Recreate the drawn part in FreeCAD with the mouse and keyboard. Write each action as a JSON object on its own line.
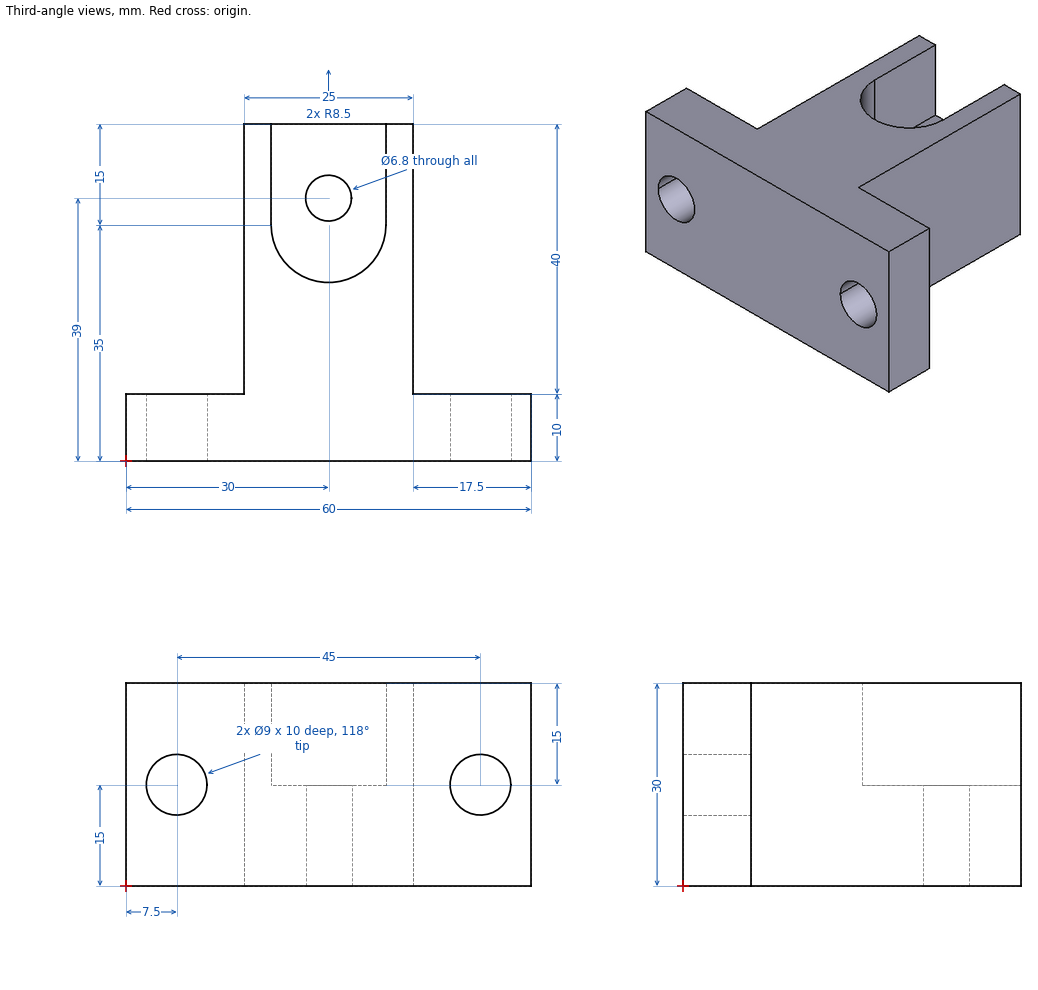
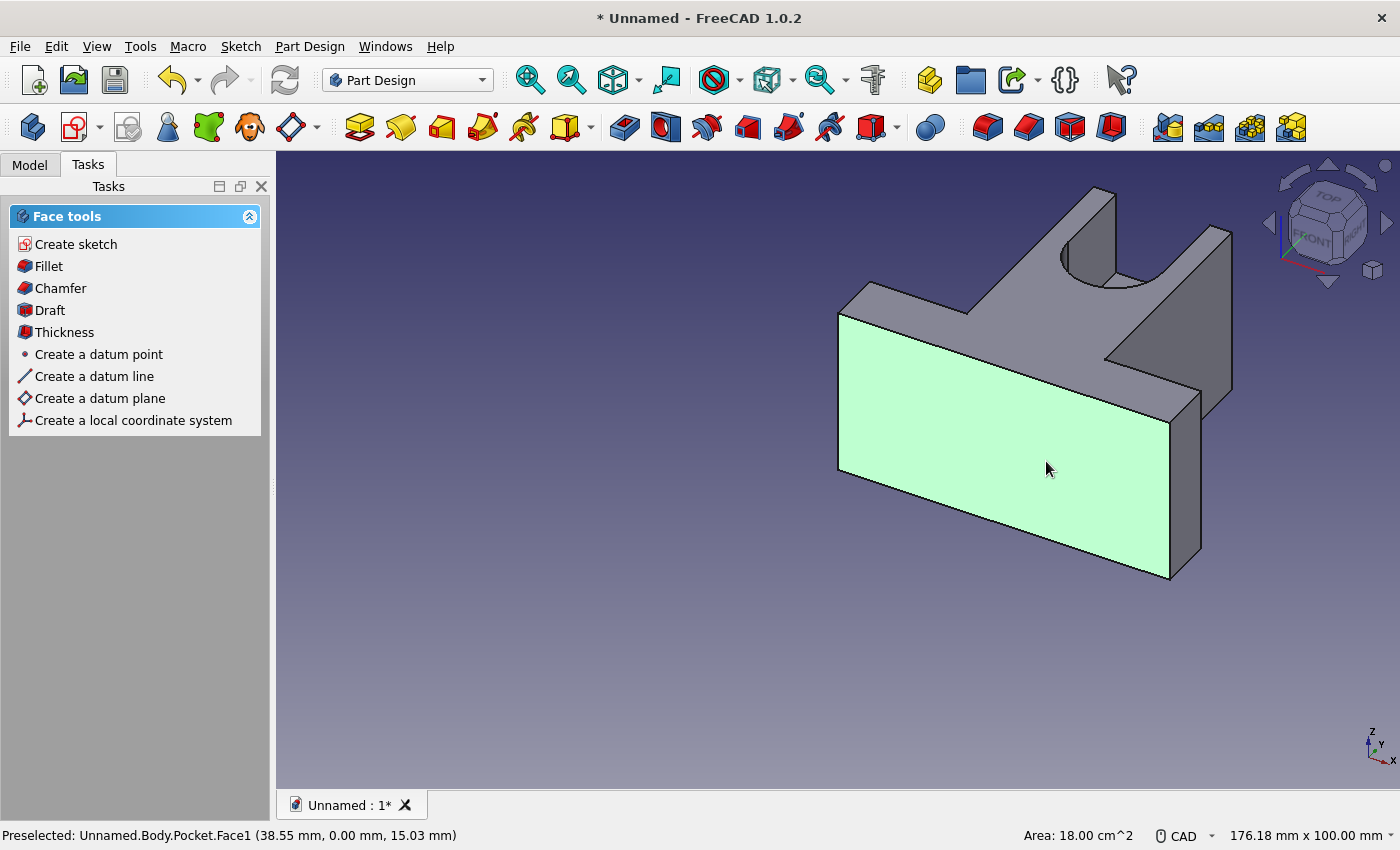
{"action": "left_click", "coordinate": [74, 128]}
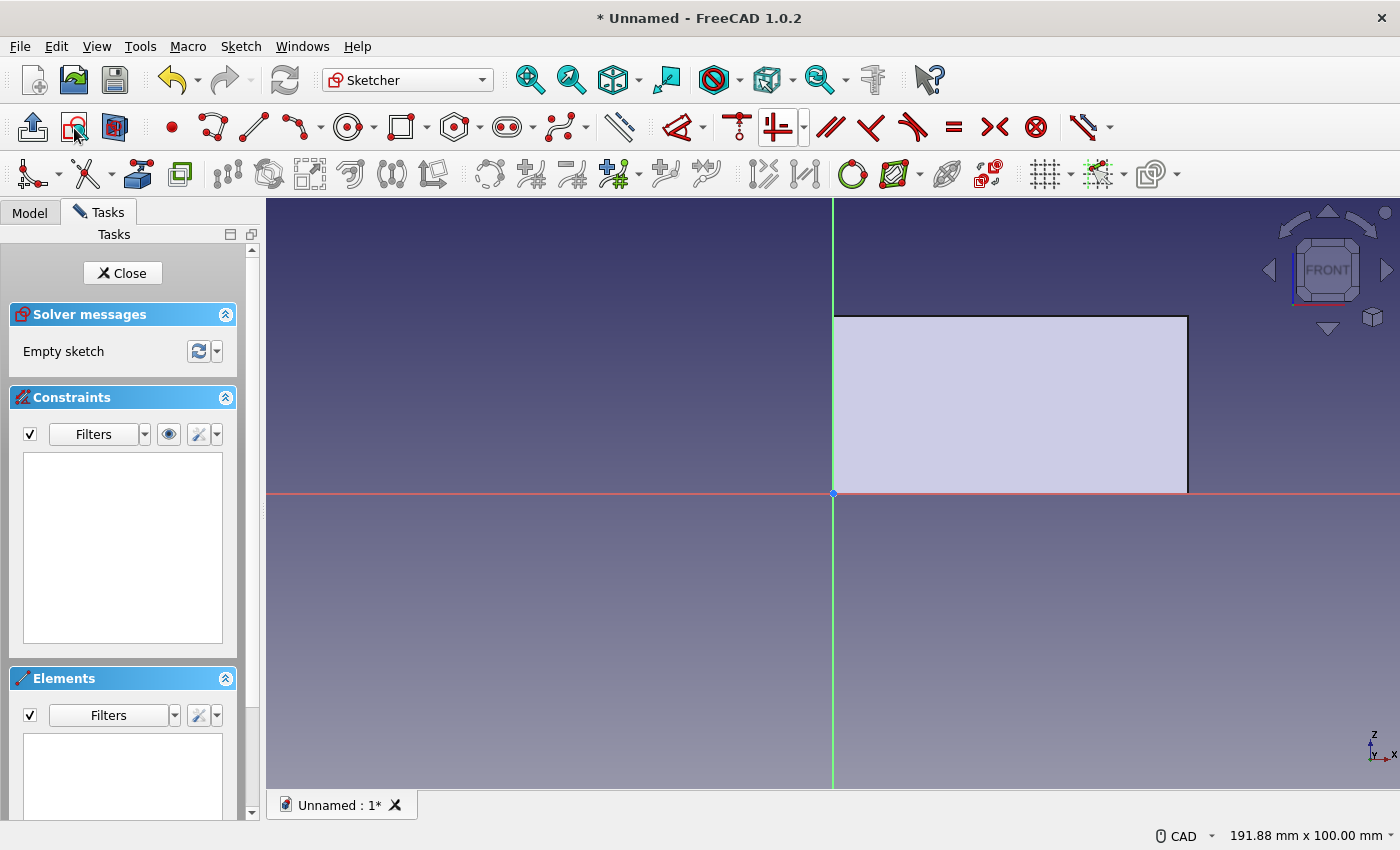
{"action": "scroll", "coordinate": [1235, 366], "scroll_direction": "up", "scroll_amount": 3}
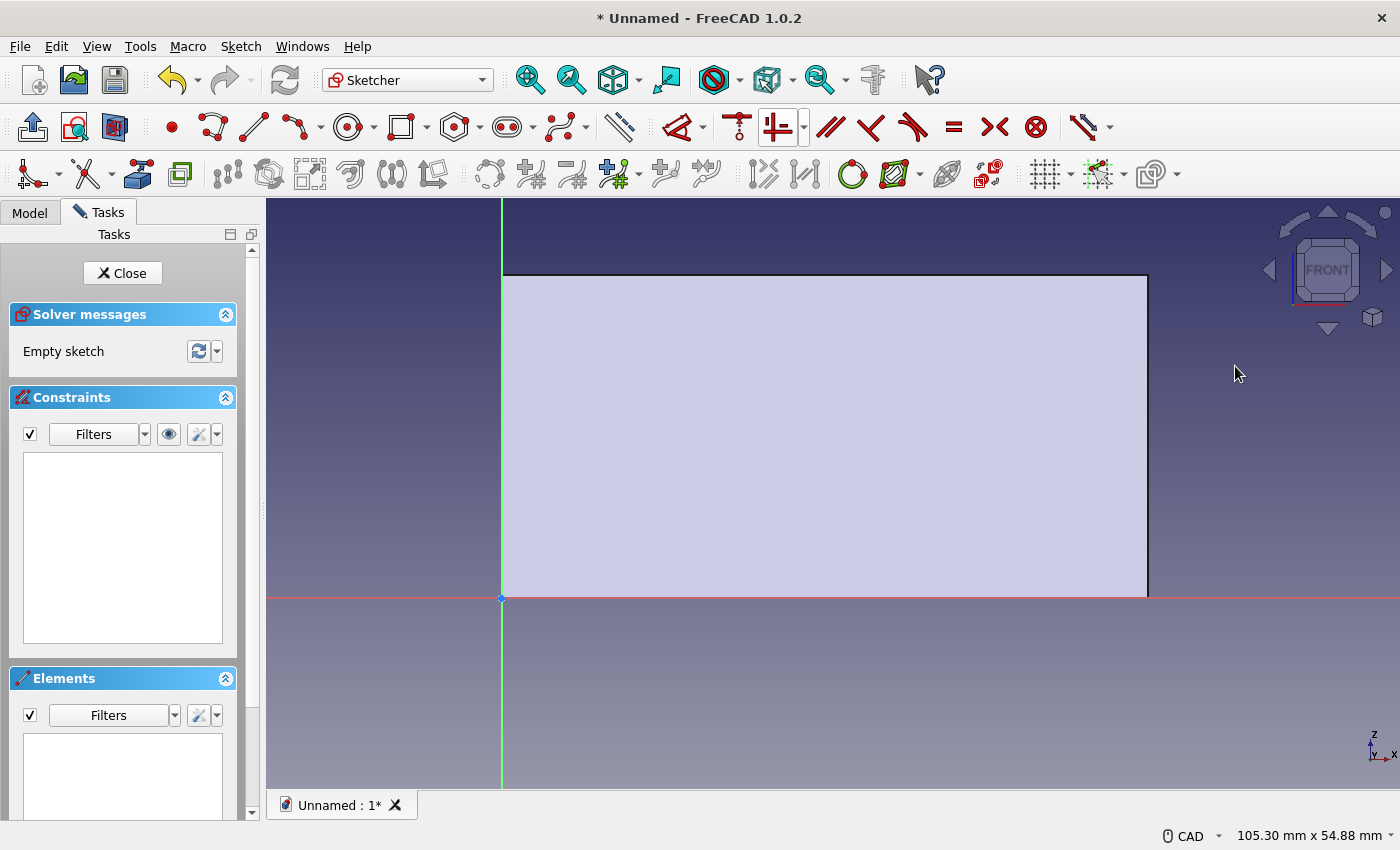
{"action": "left_click", "coordinate": [348, 128]}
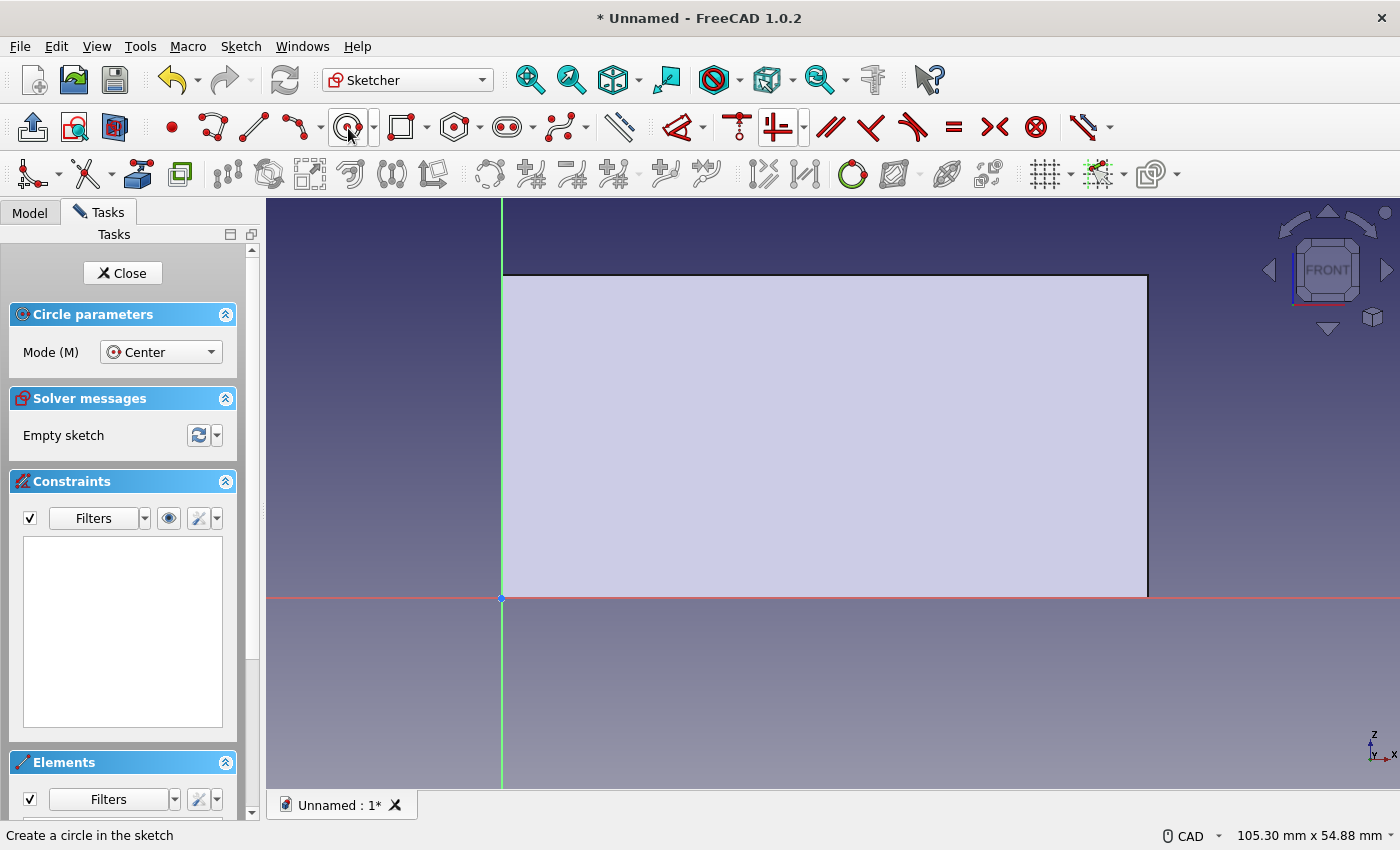
{"action": "left_click", "coordinate": [583, 437]}
{"action": "left_click", "coordinate": [617, 402]}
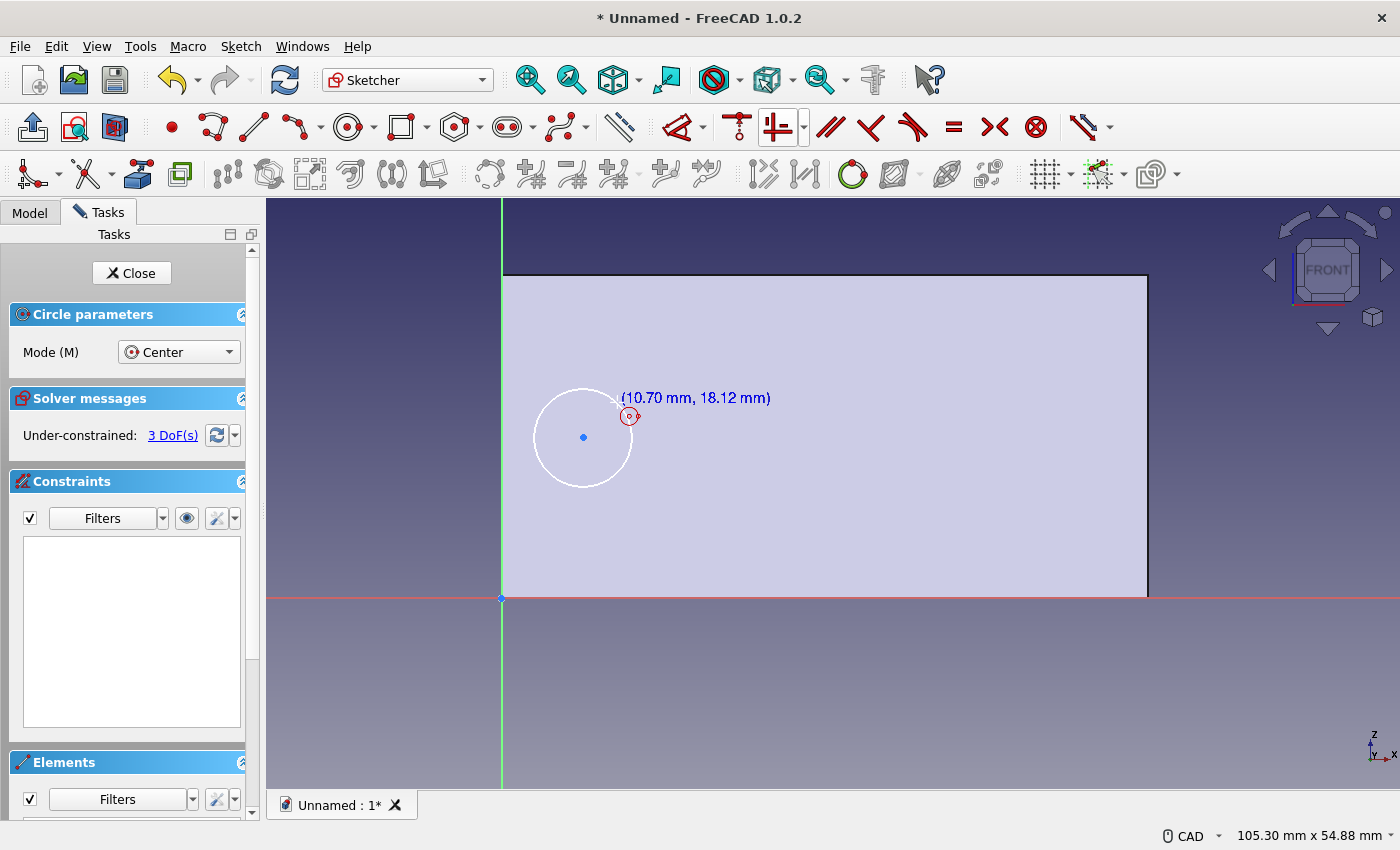
{"action": "left_click", "coordinate": [1067, 437]}
{"action": "left_click", "coordinate": [1101, 402]}
{"action": "key", "text": "Escape"}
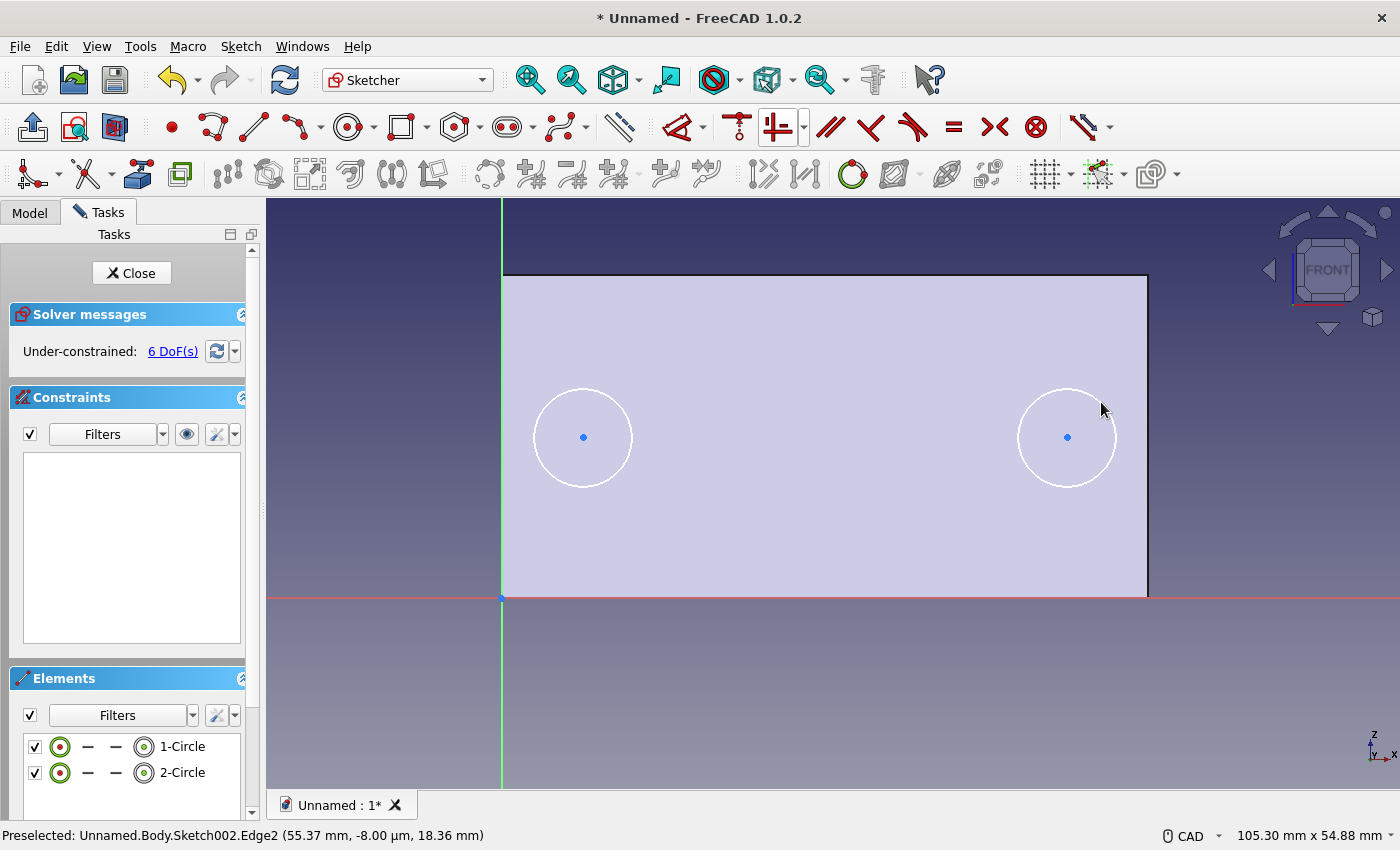
{"action": "left_click", "coordinate": [617, 403]}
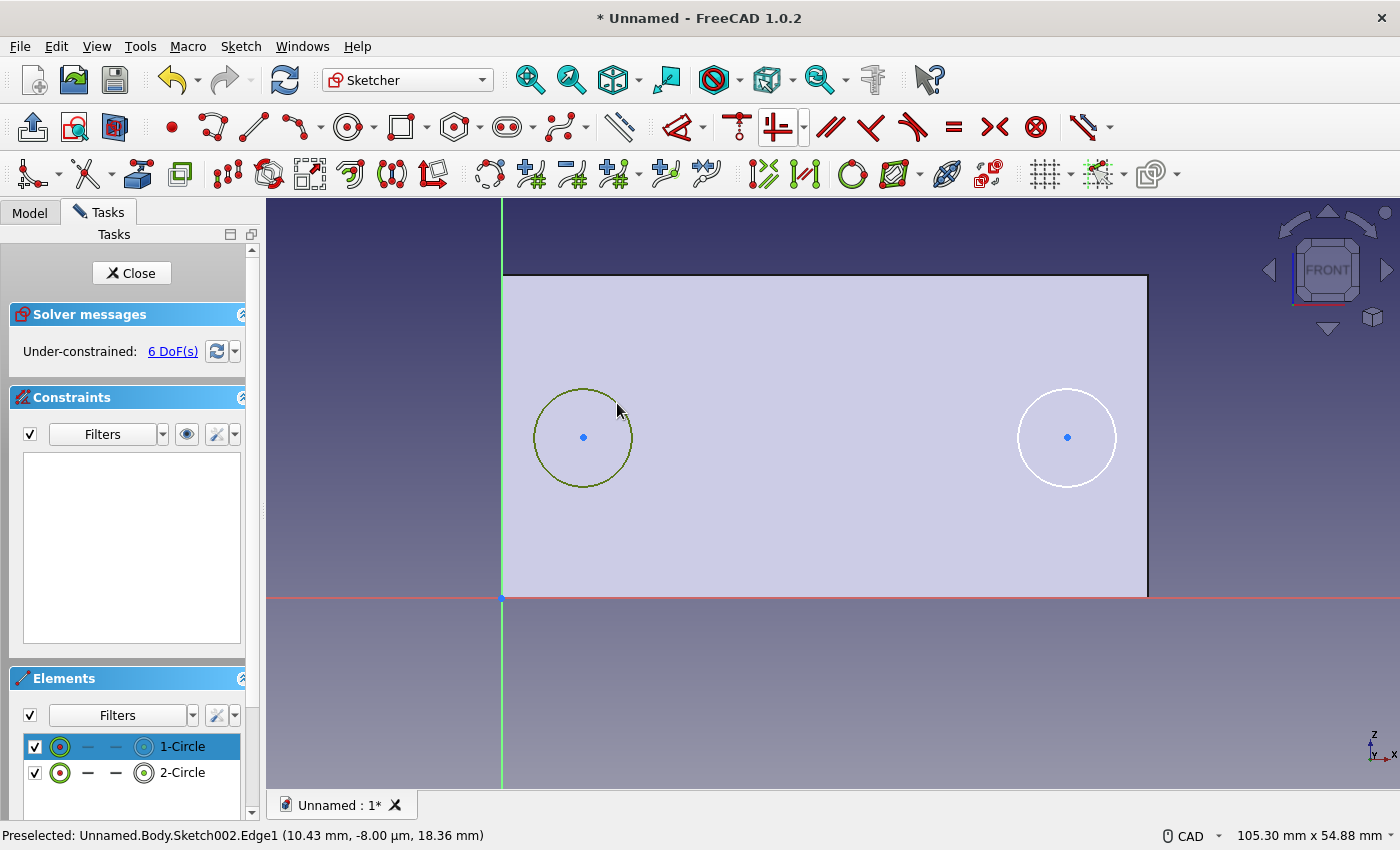
{"action": "left_click", "coordinate": [1101, 403]}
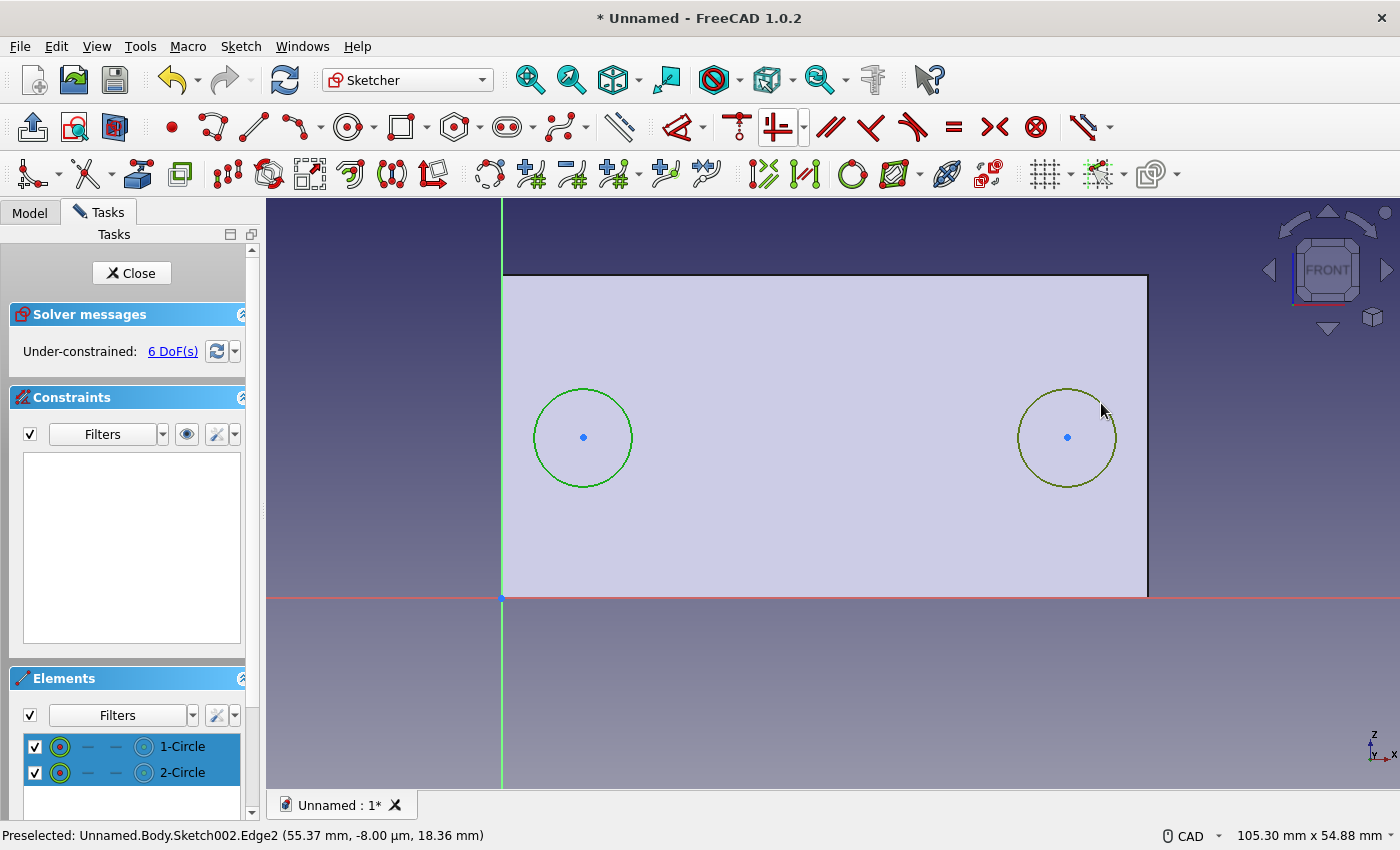
{"action": "left_click", "coordinate": [954, 128]}